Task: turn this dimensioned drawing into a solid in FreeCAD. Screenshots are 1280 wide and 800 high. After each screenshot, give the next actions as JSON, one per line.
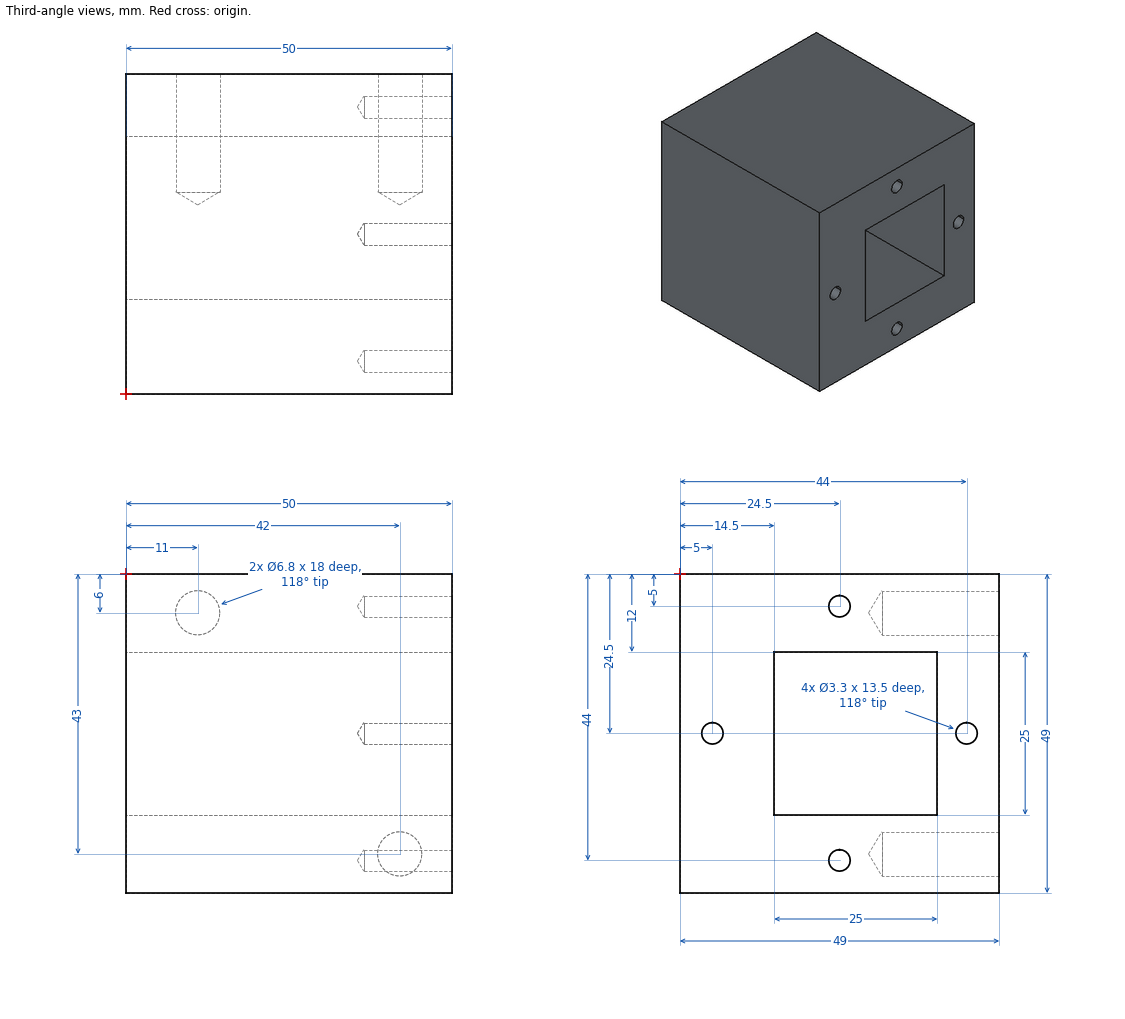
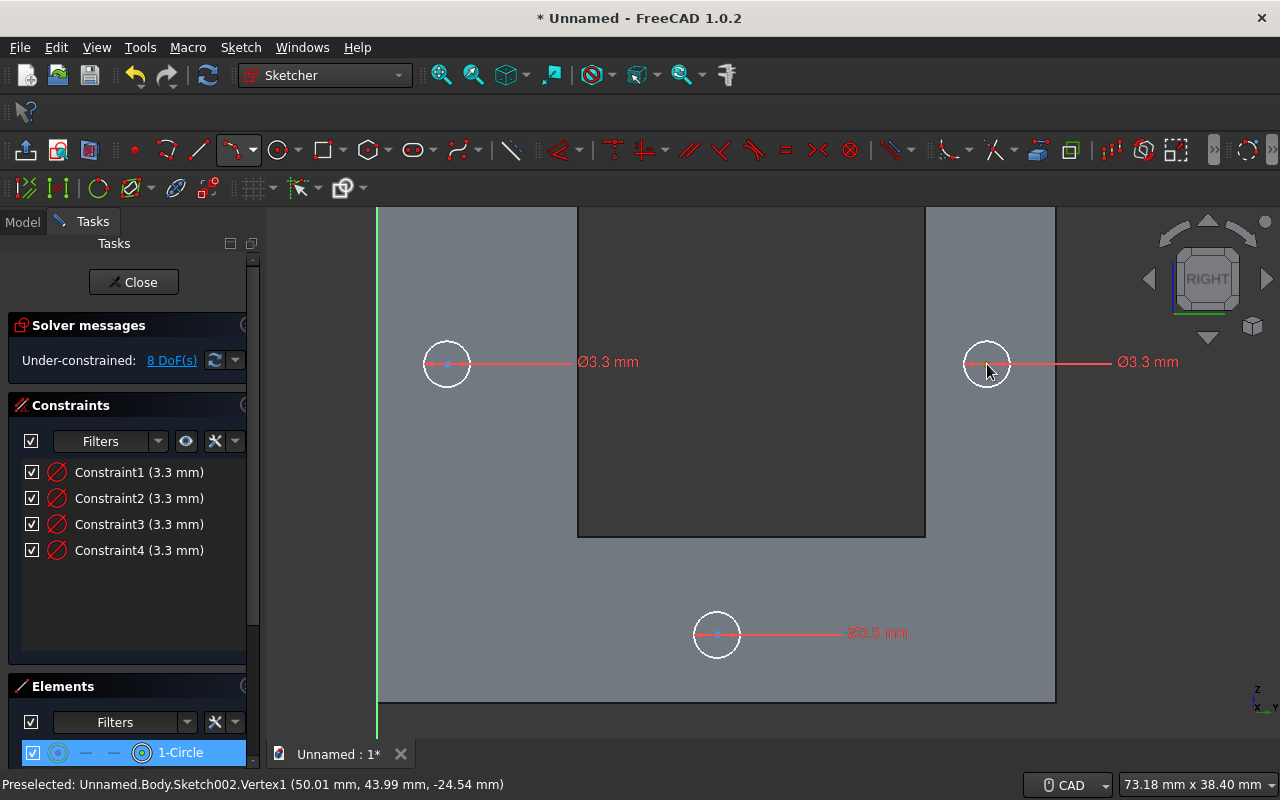
{"action": "left_click", "coordinate": [447, 364]}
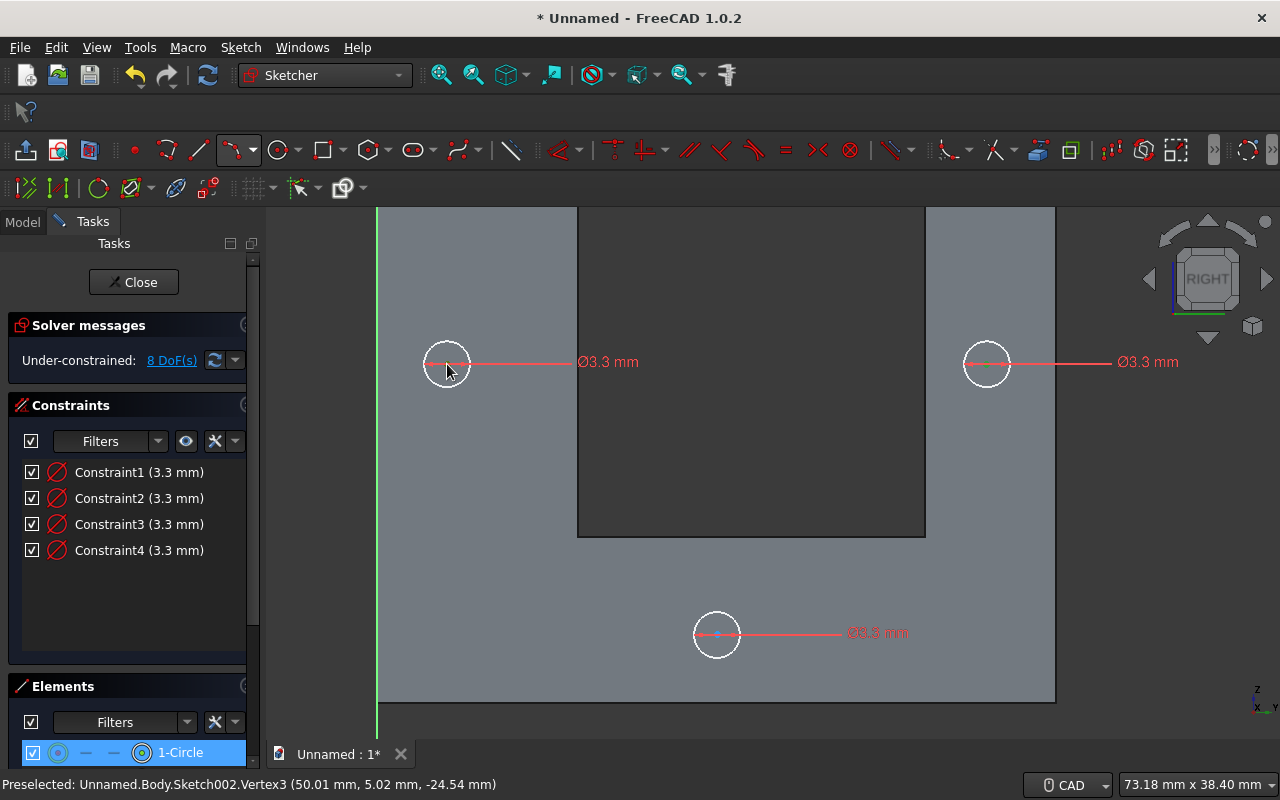
{"action": "key", "text": "h"}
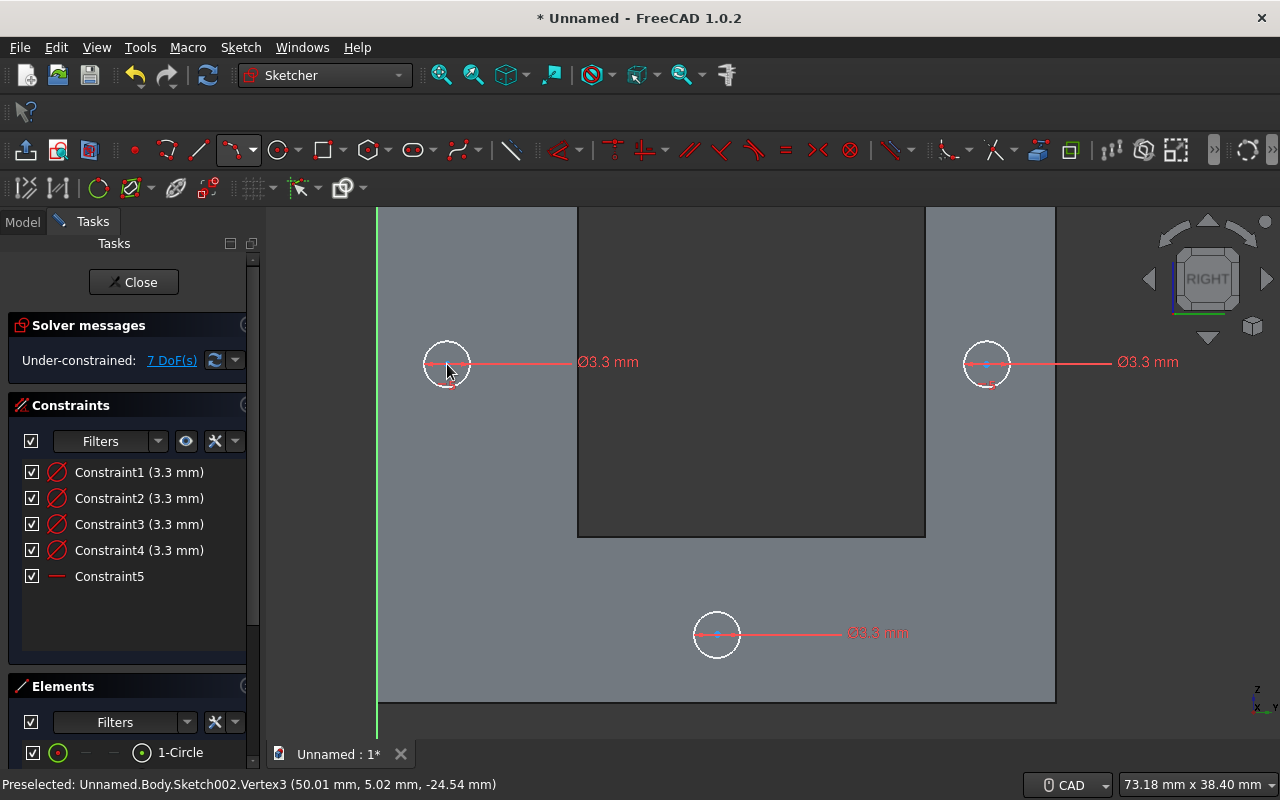
{"action": "scroll", "coordinate": [718, 634], "scroll_direction": "down", "scroll_amount": 3}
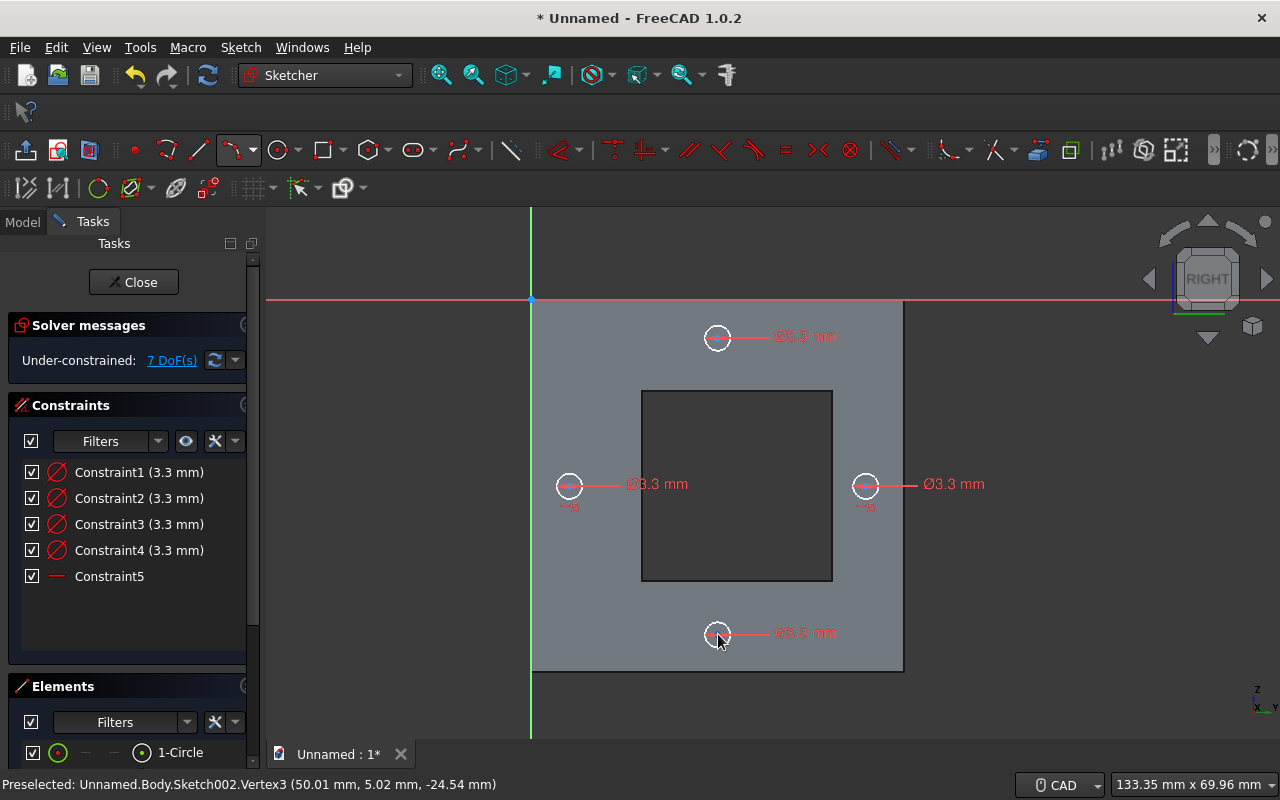
{"action": "left_click", "coordinate": [718, 338]}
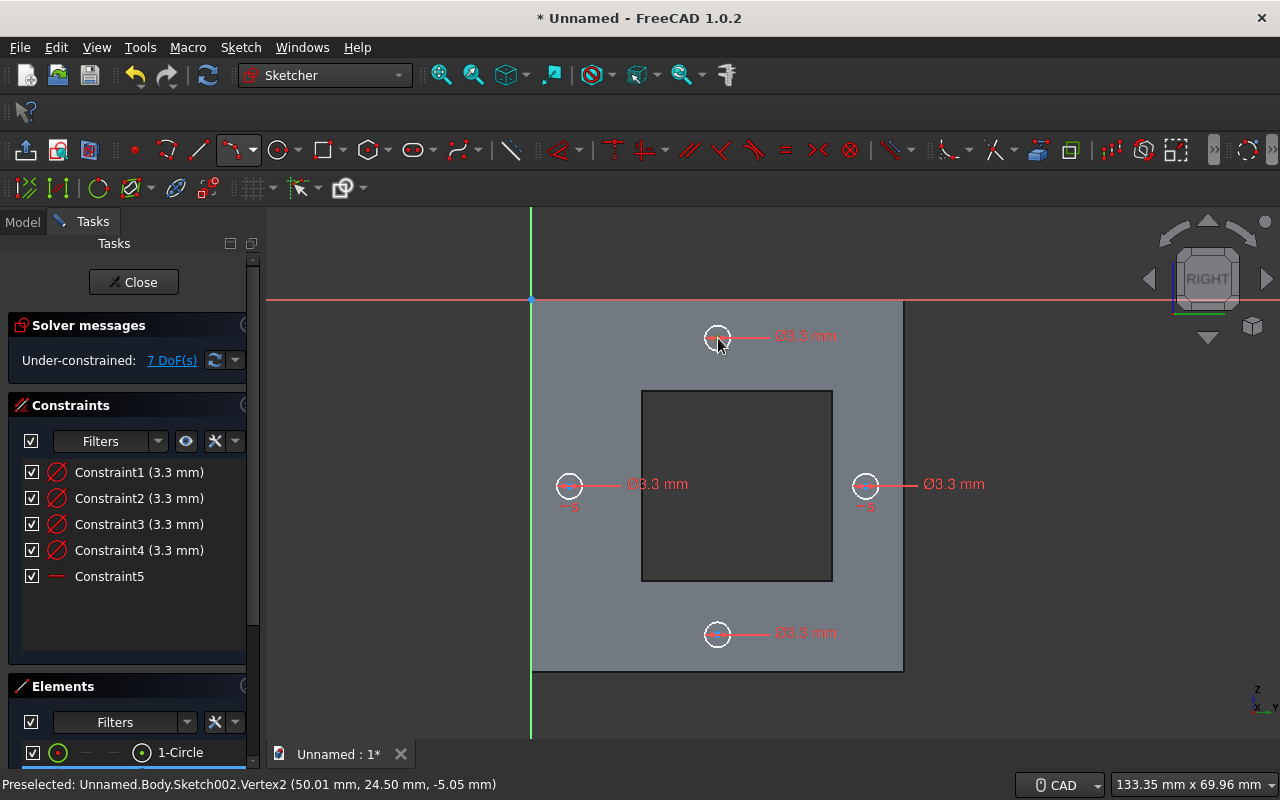
{"action": "left_click", "coordinate": [718, 635]}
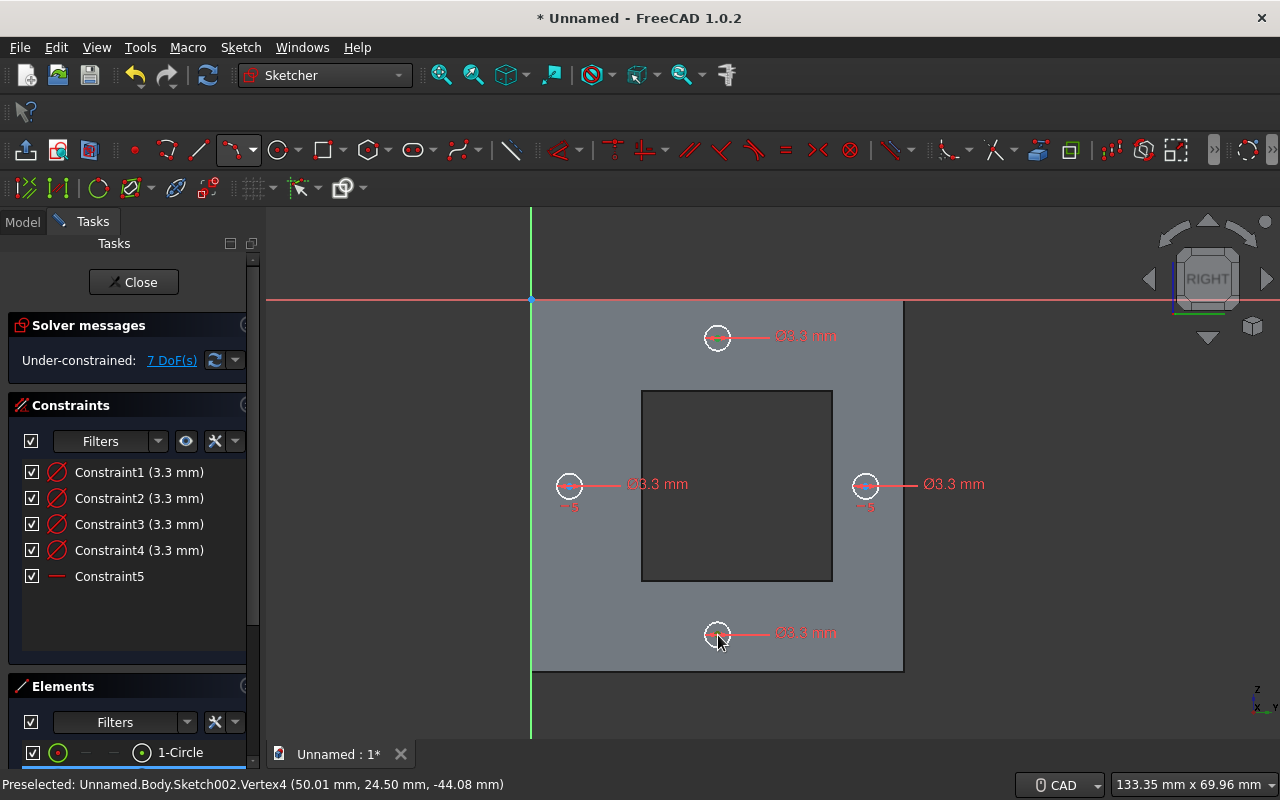
{"action": "key", "text": "v"}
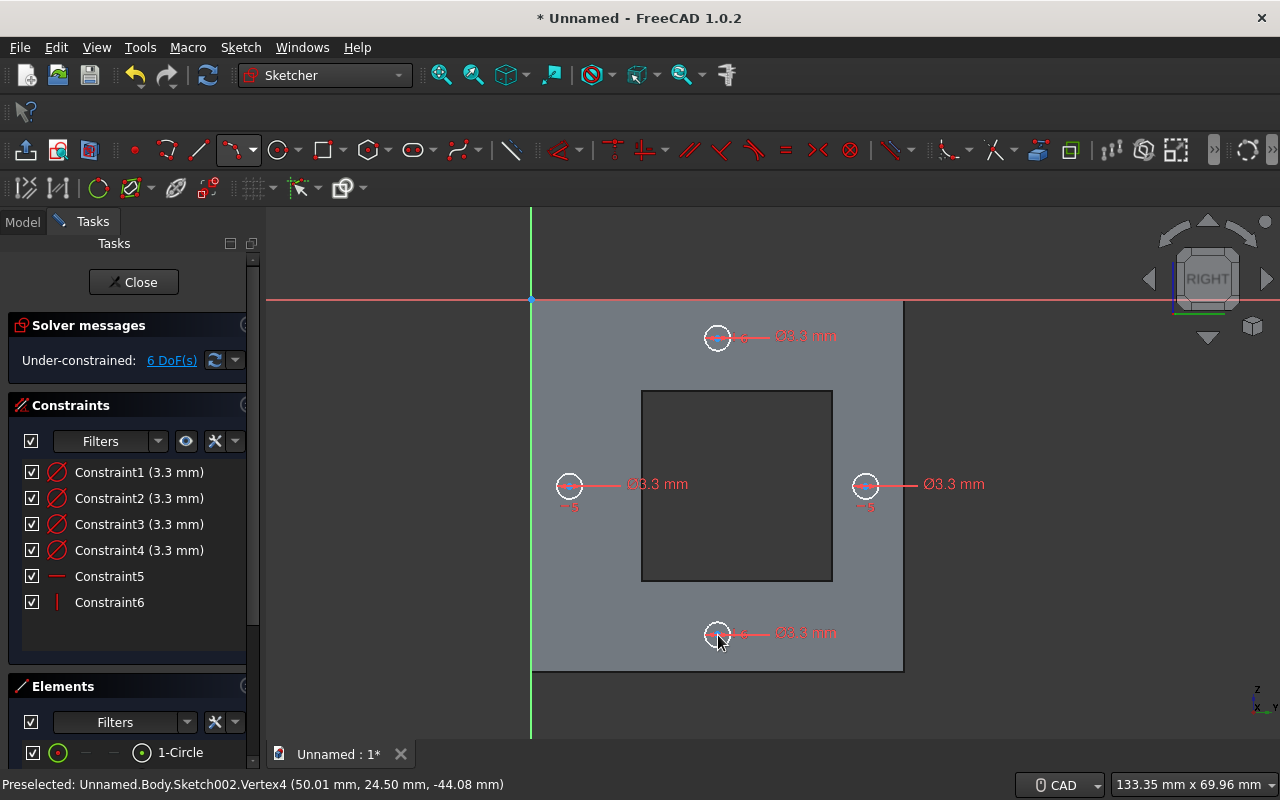
{"action": "key", "text": "d"}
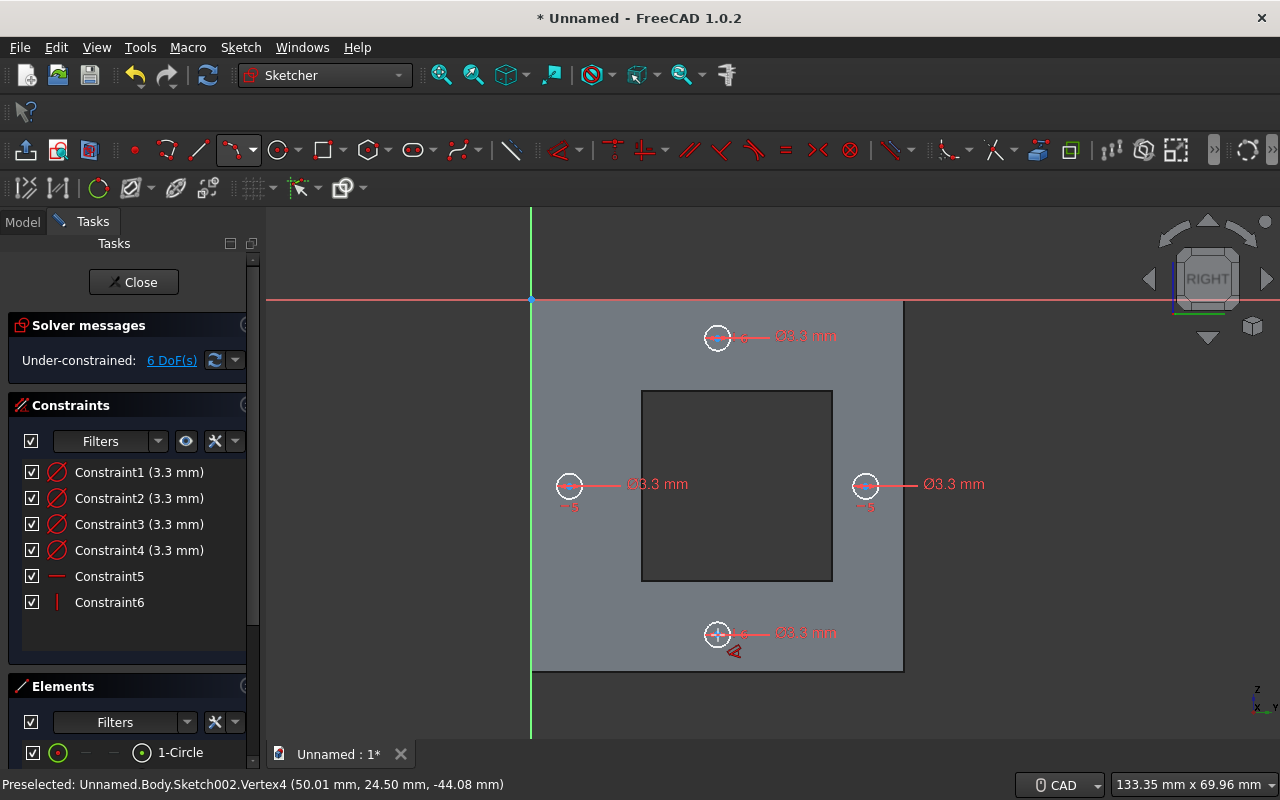
{"action": "left_click", "coordinate": [718, 338]}
{"action": "left_click", "coordinate": [497, 319]}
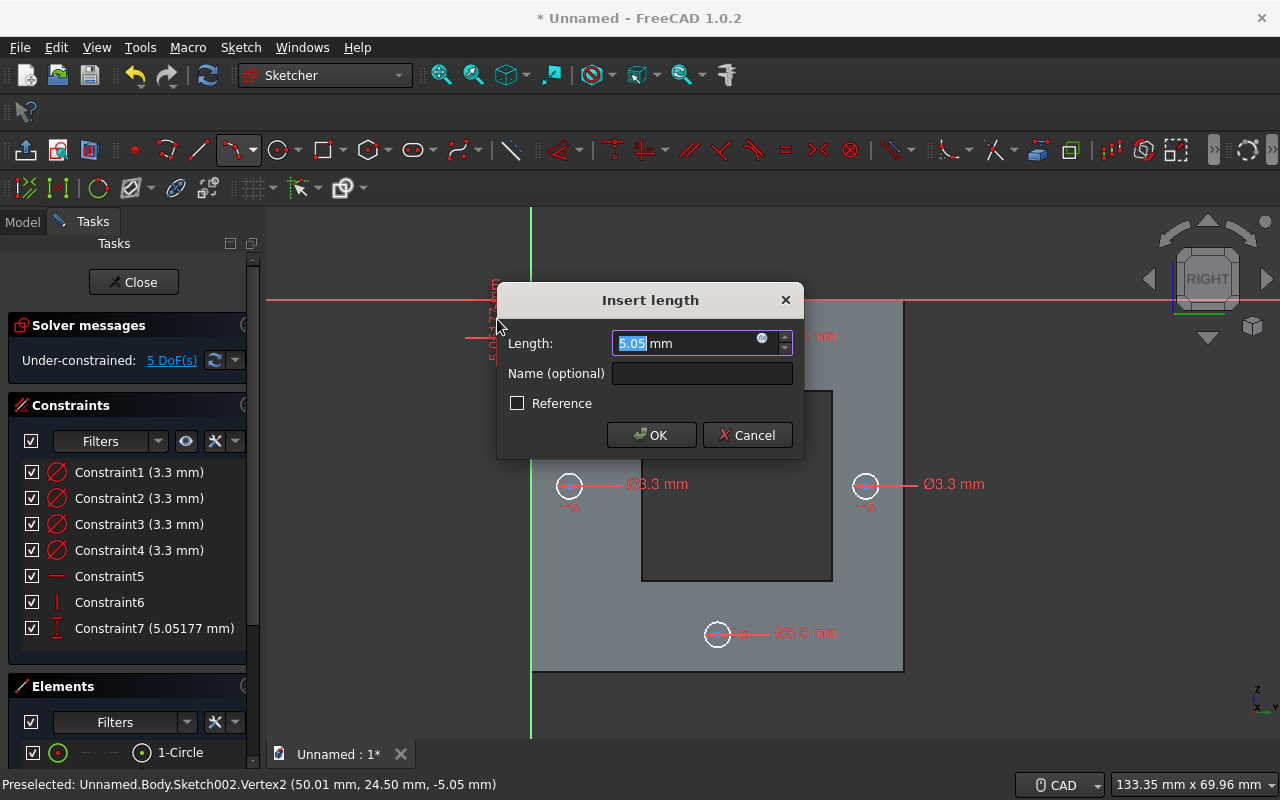
{"action": "type", "text": "5"}
{"action": "key", "text": "Return"}